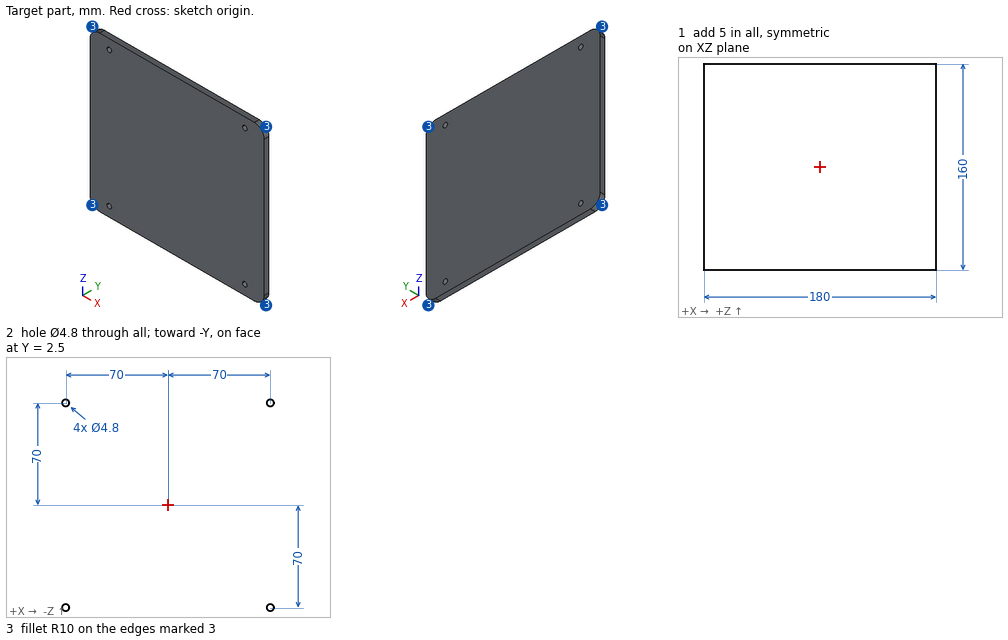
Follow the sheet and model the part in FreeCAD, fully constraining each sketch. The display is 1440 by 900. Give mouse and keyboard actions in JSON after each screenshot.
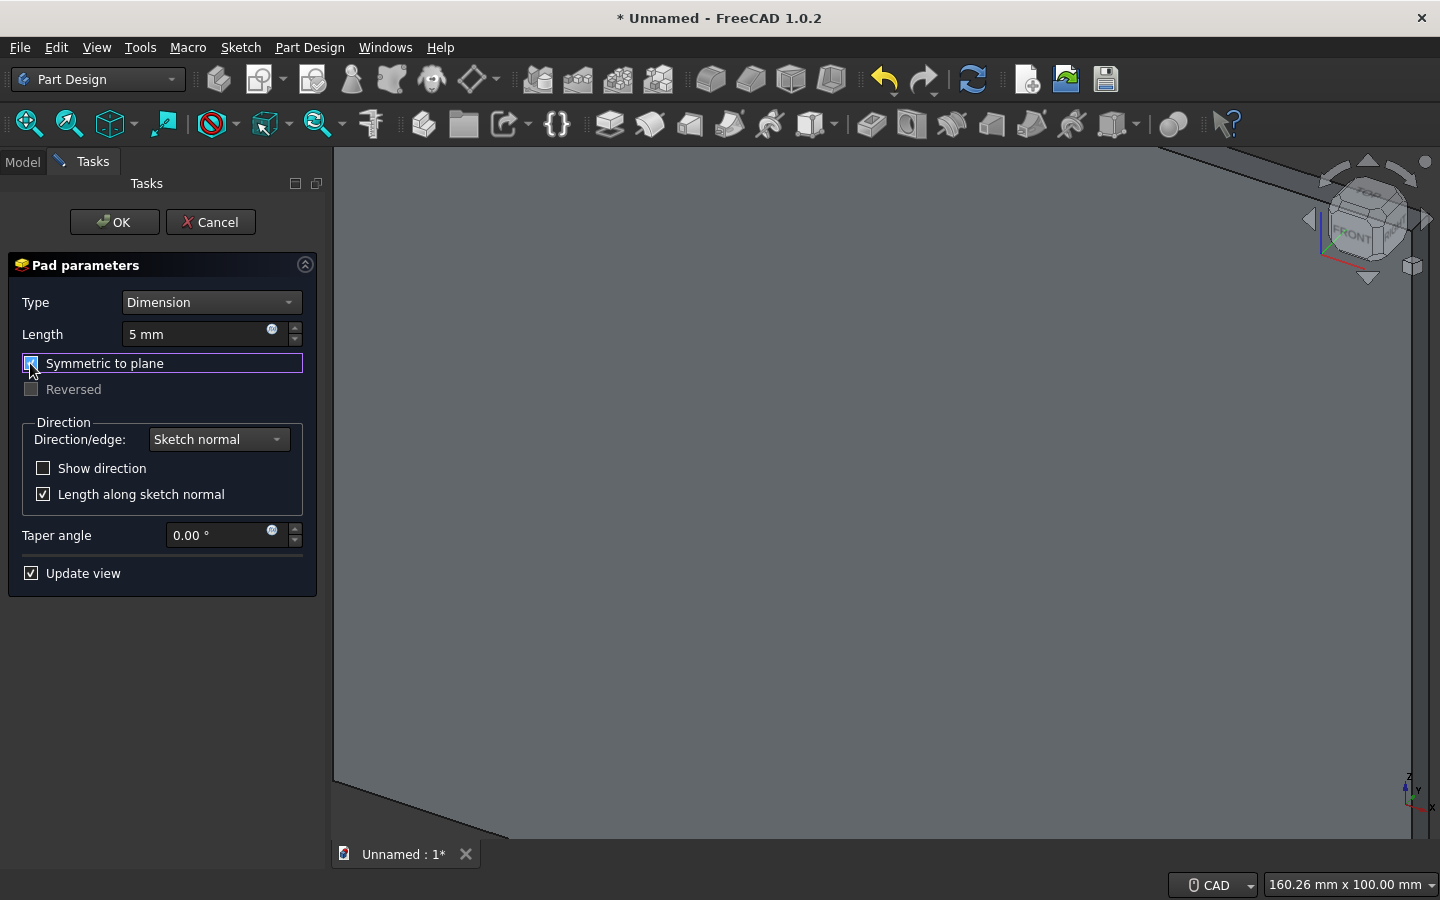
{"action": "left_click", "coordinate": [115, 222]}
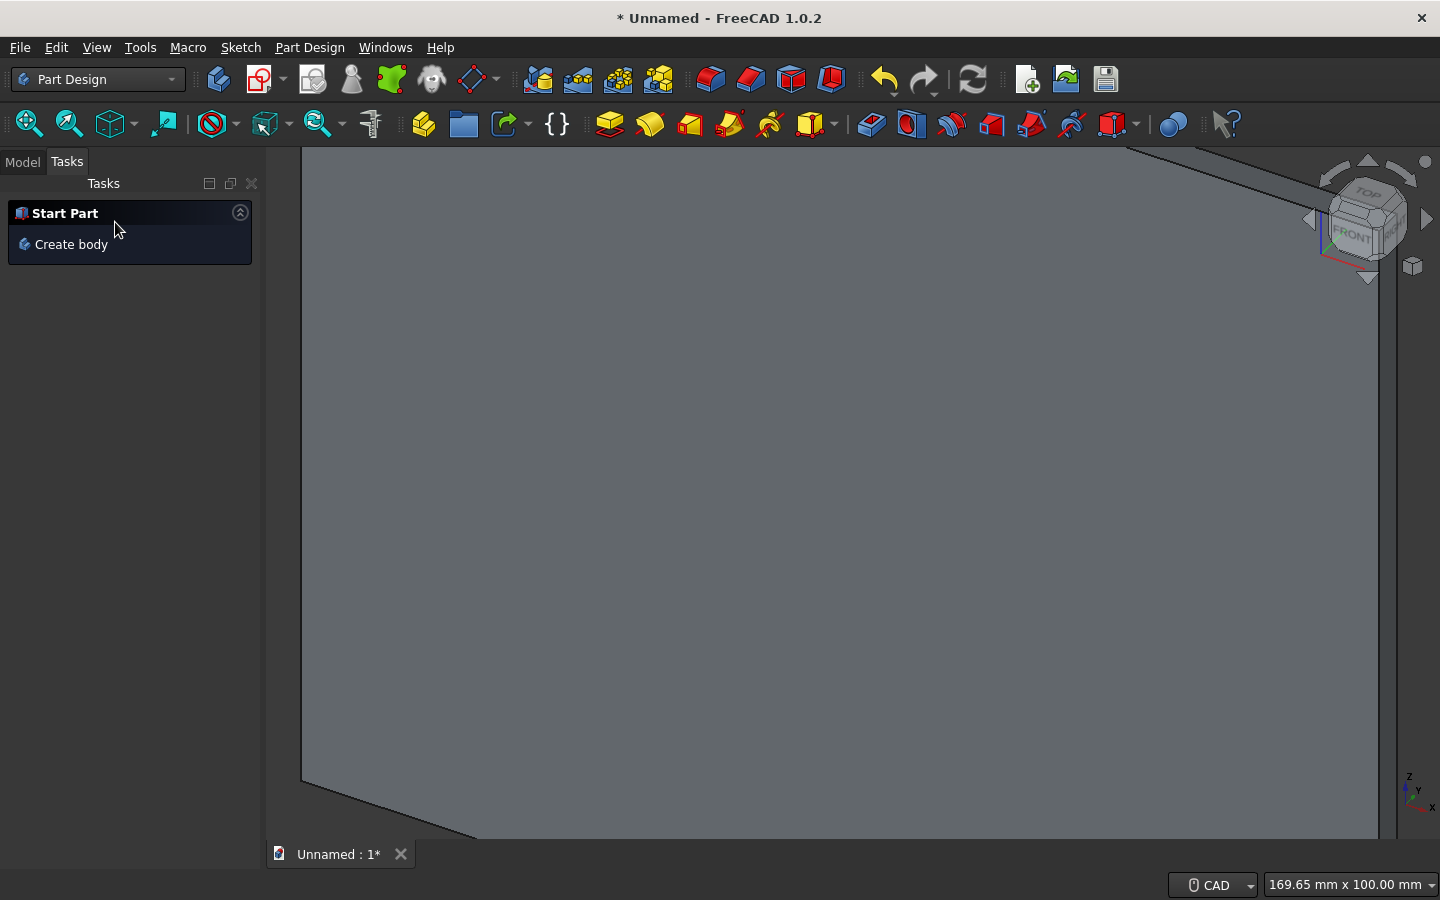
{"action": "left_click", "coordinate": [30, 124]}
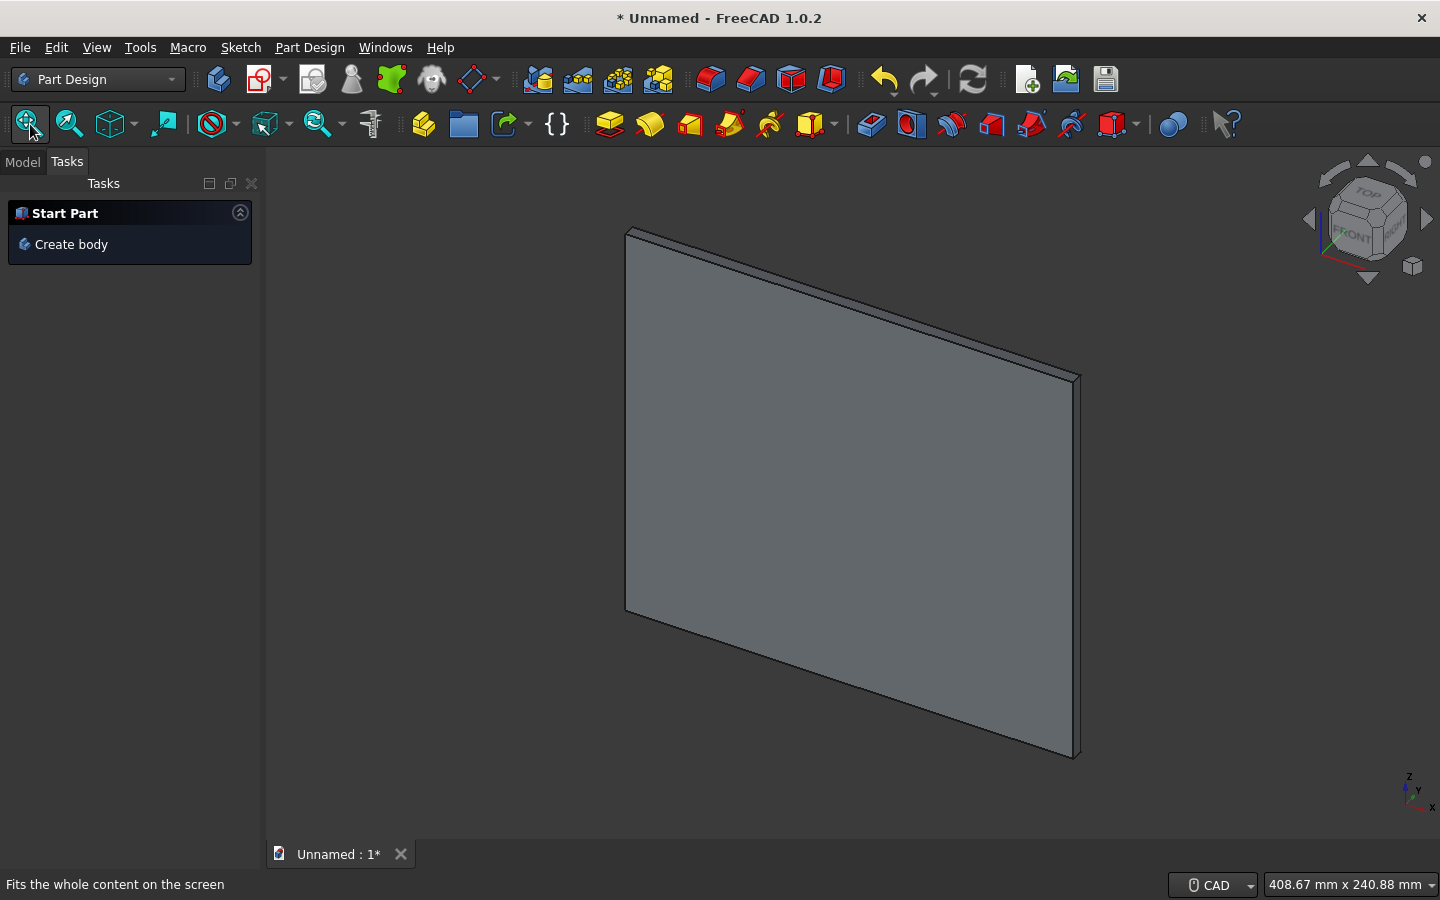
{"action": "key", "text": "4"}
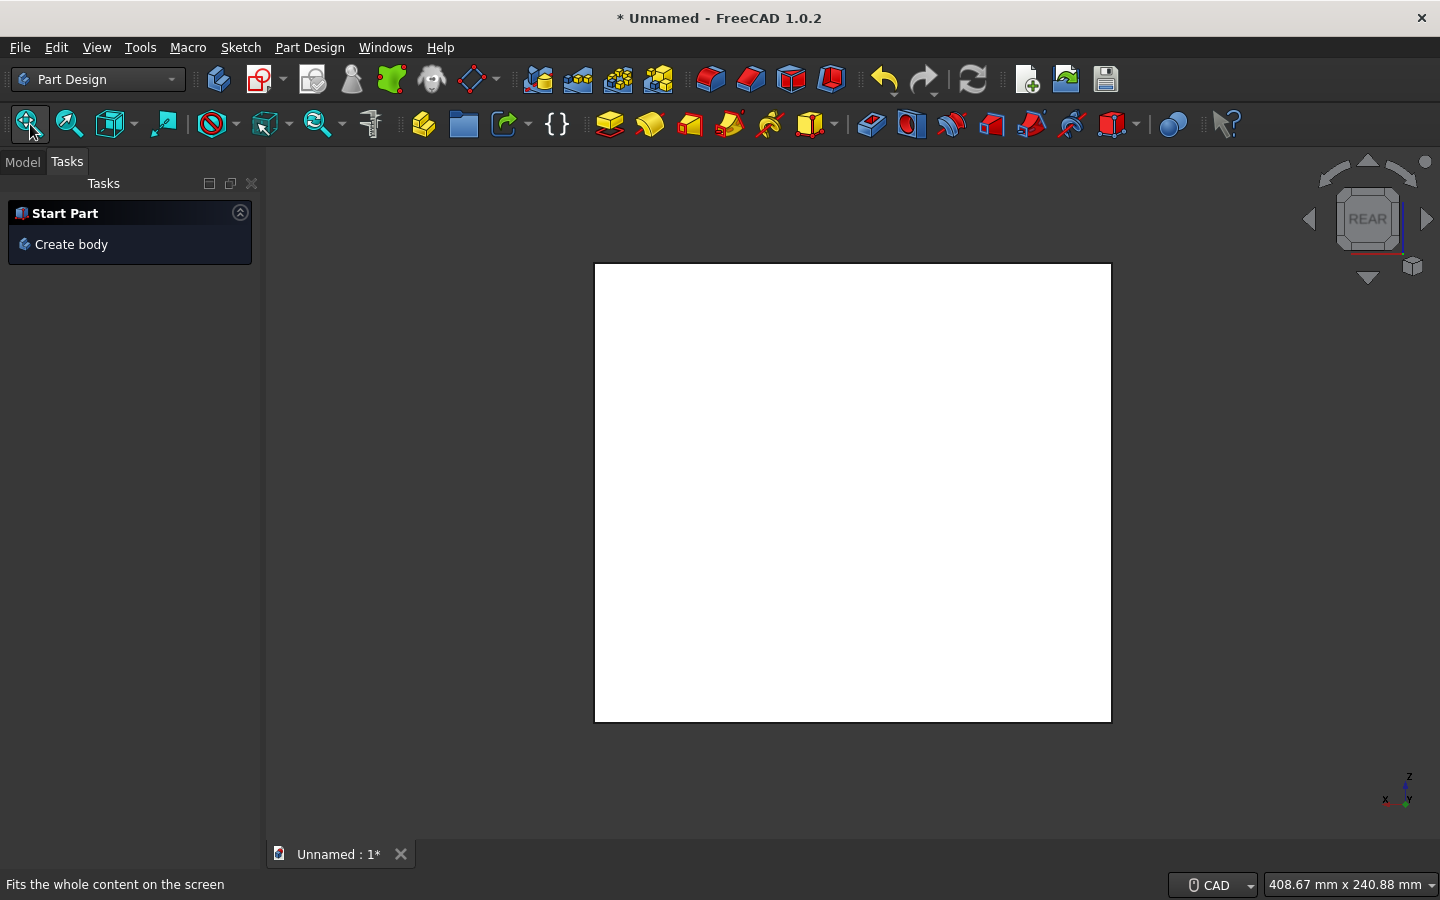
{"action": "left_click", "coordinate": [853, 492]}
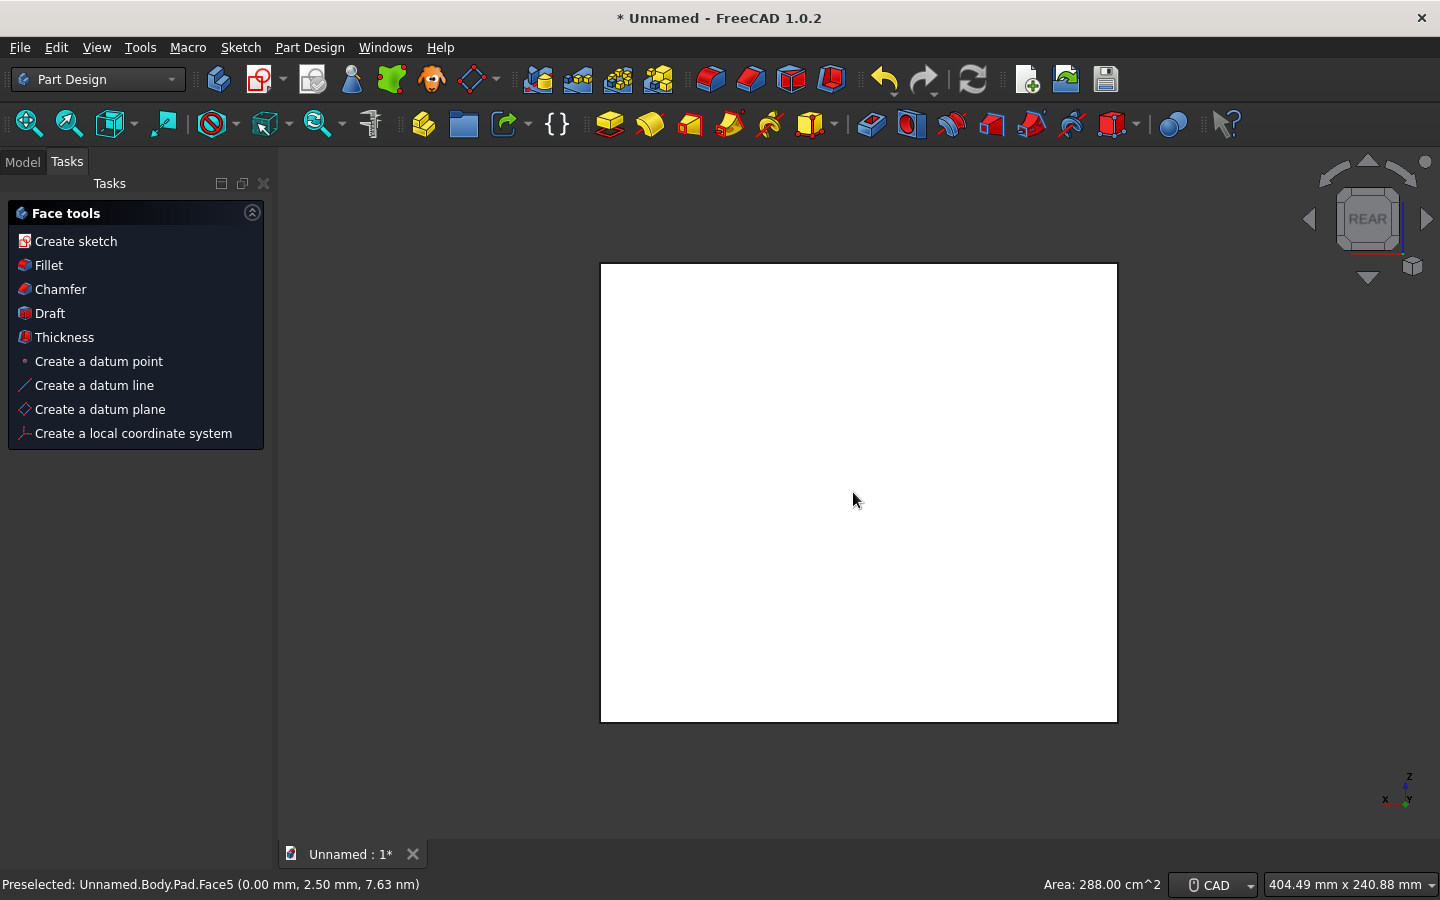
{"action": "left_click", "coordinate": [260, 80]}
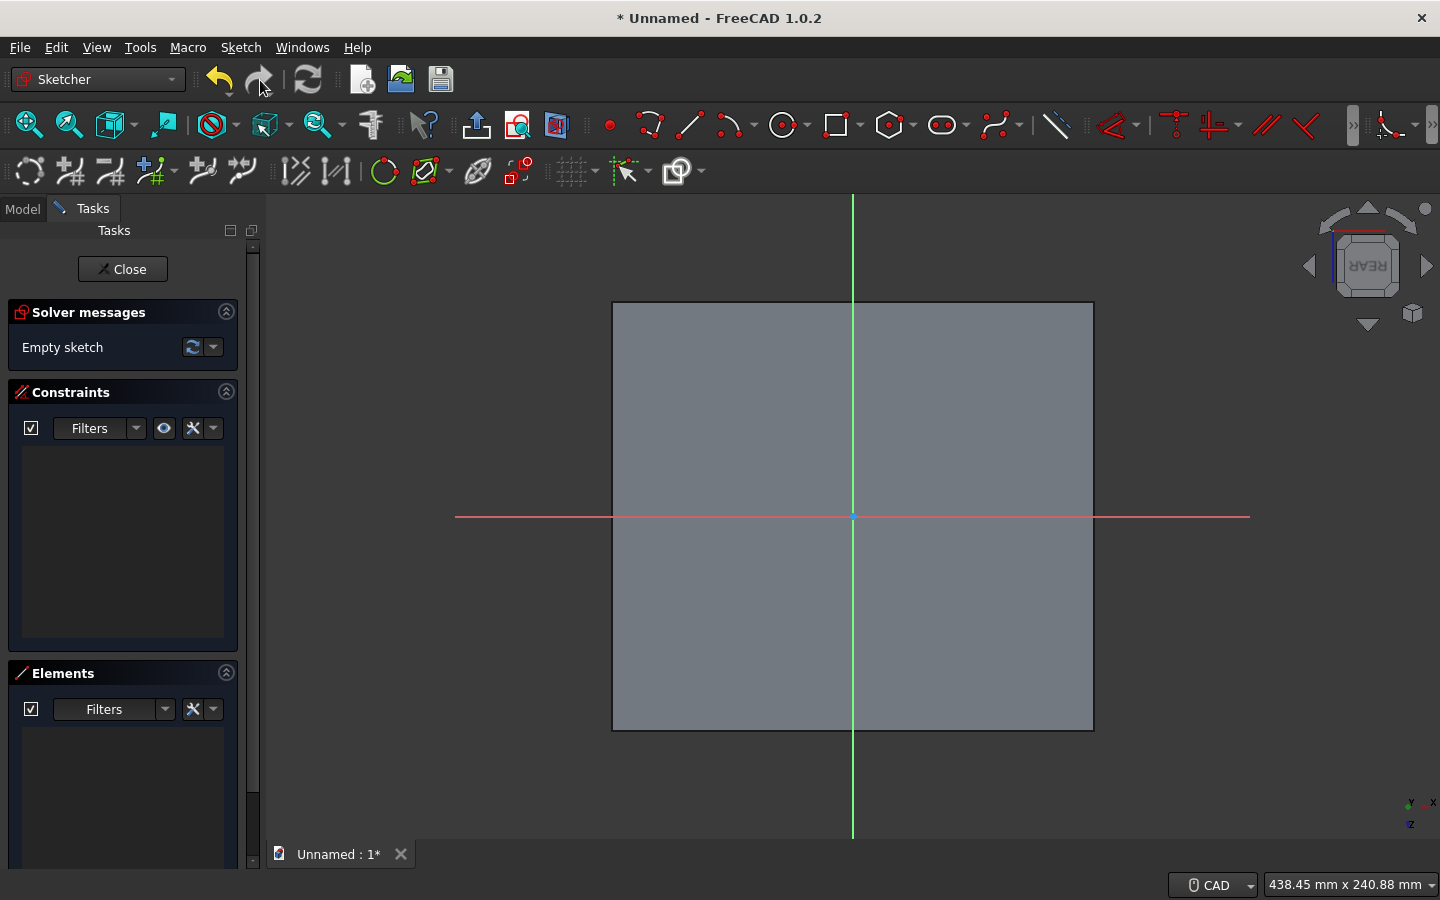
{"action": "left_click", "coordinate": [784, 126]}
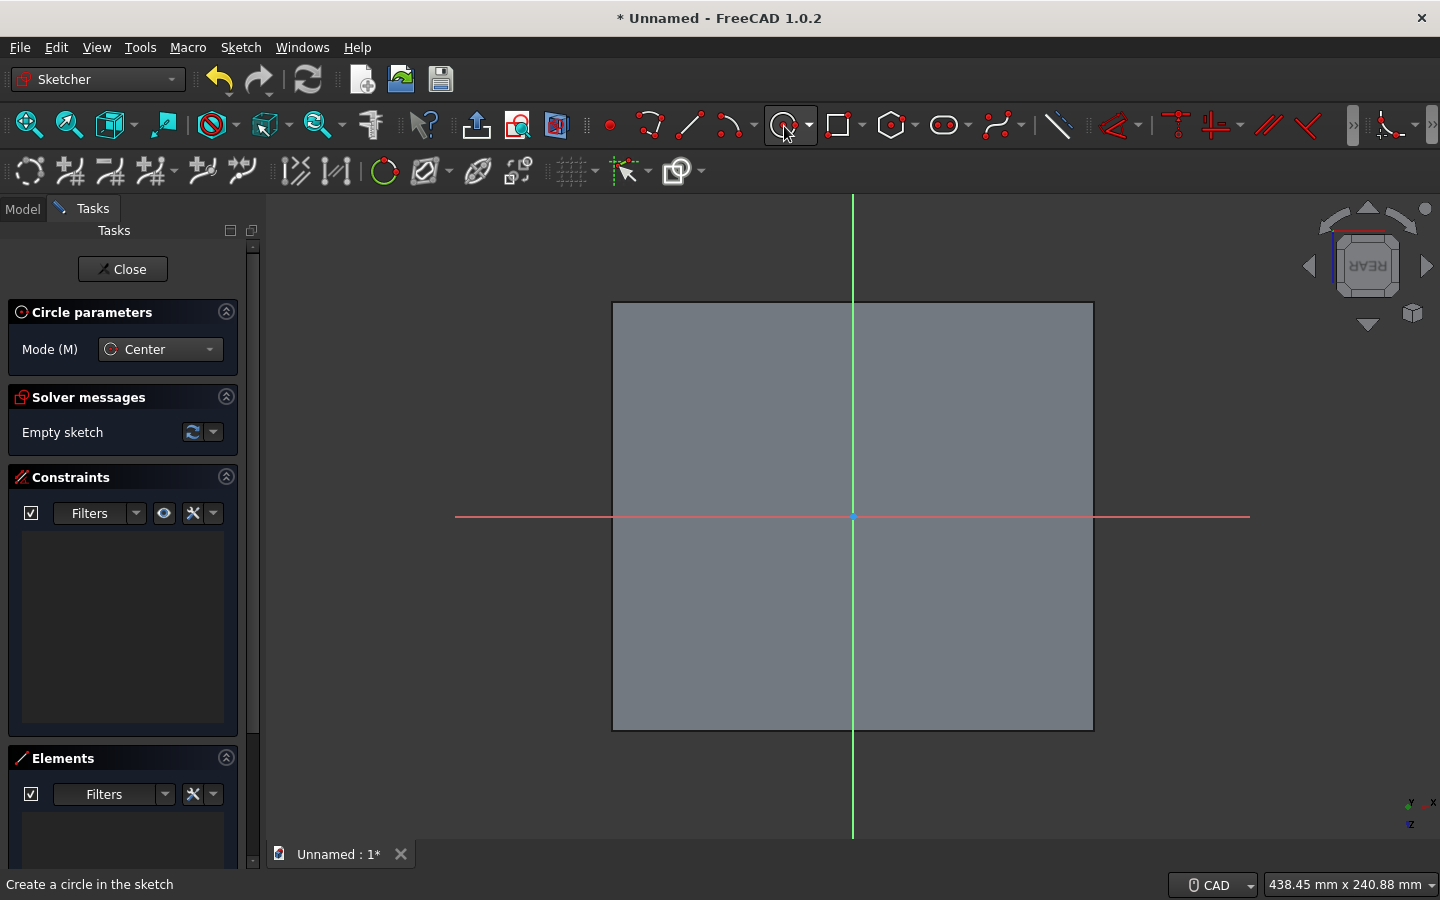
{"action": "scroll", "coordinate": [666, 329], "scroll_direction": "up", "scroll_amount": 7}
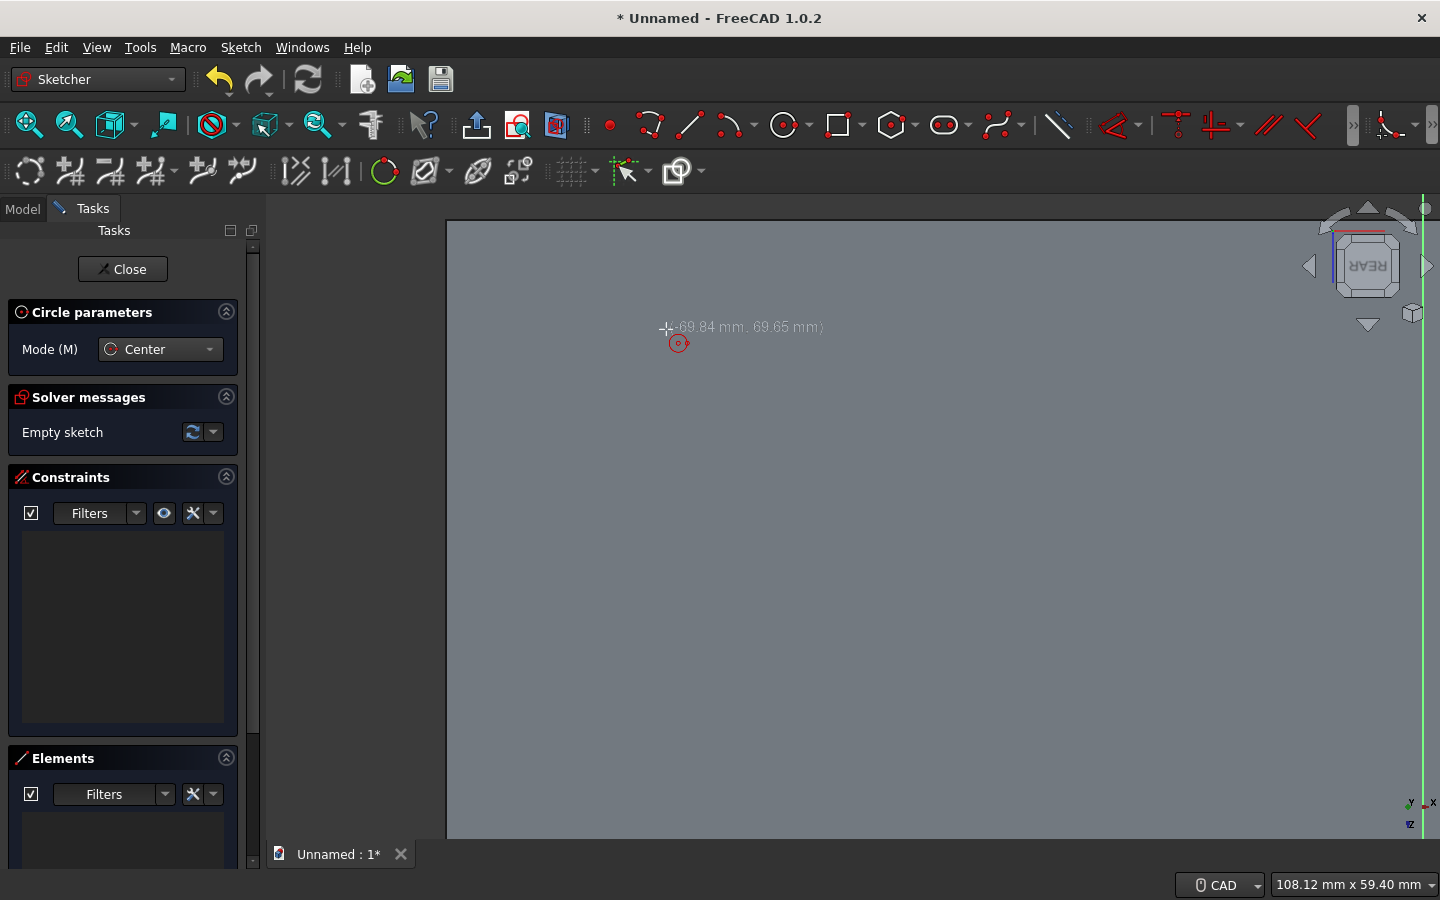
{"action": "scroll", "coordinate": [575, 329], "scroll_direction": "down", "scroll_amount": 7}